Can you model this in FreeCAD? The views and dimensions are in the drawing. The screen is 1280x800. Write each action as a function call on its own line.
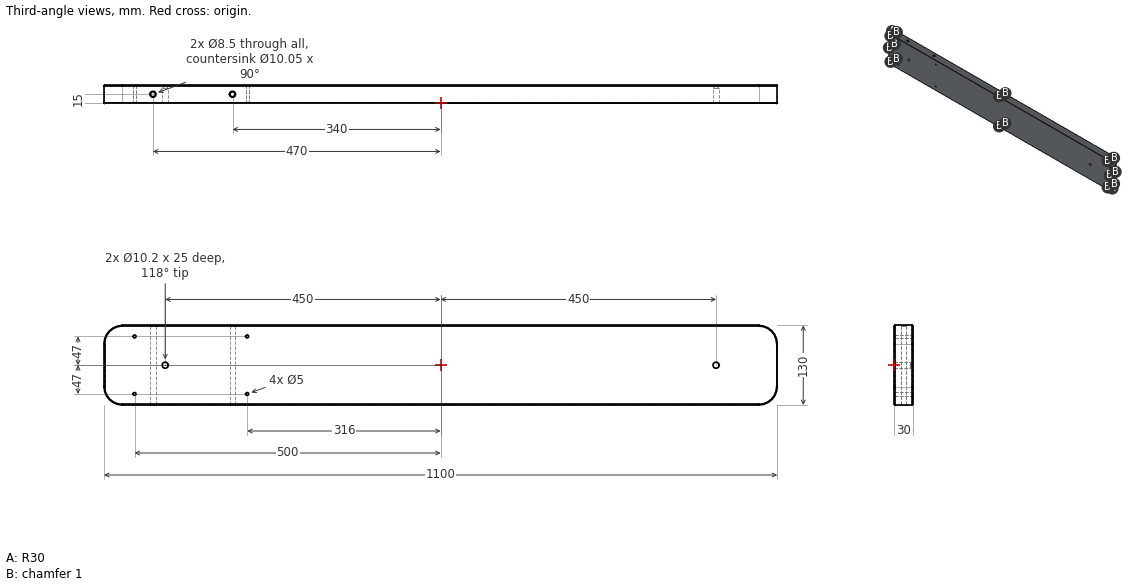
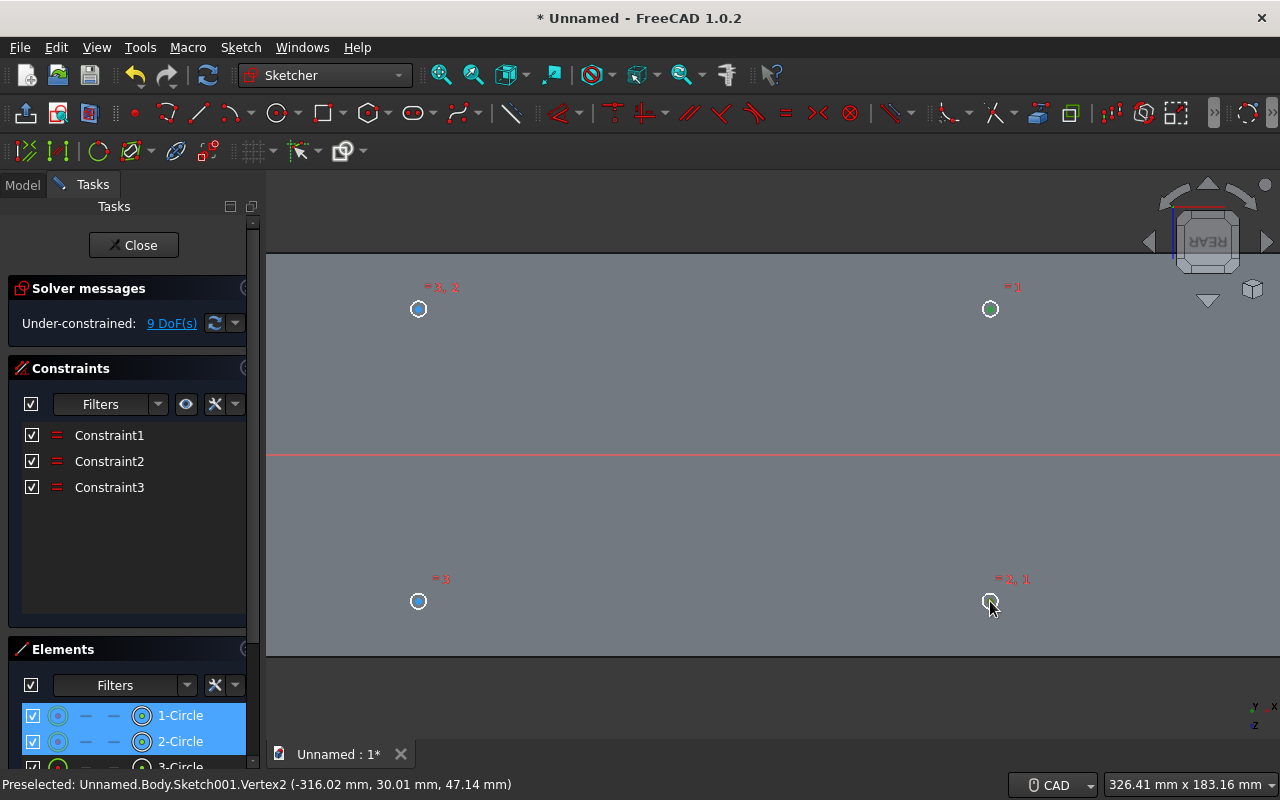
click(668, 114)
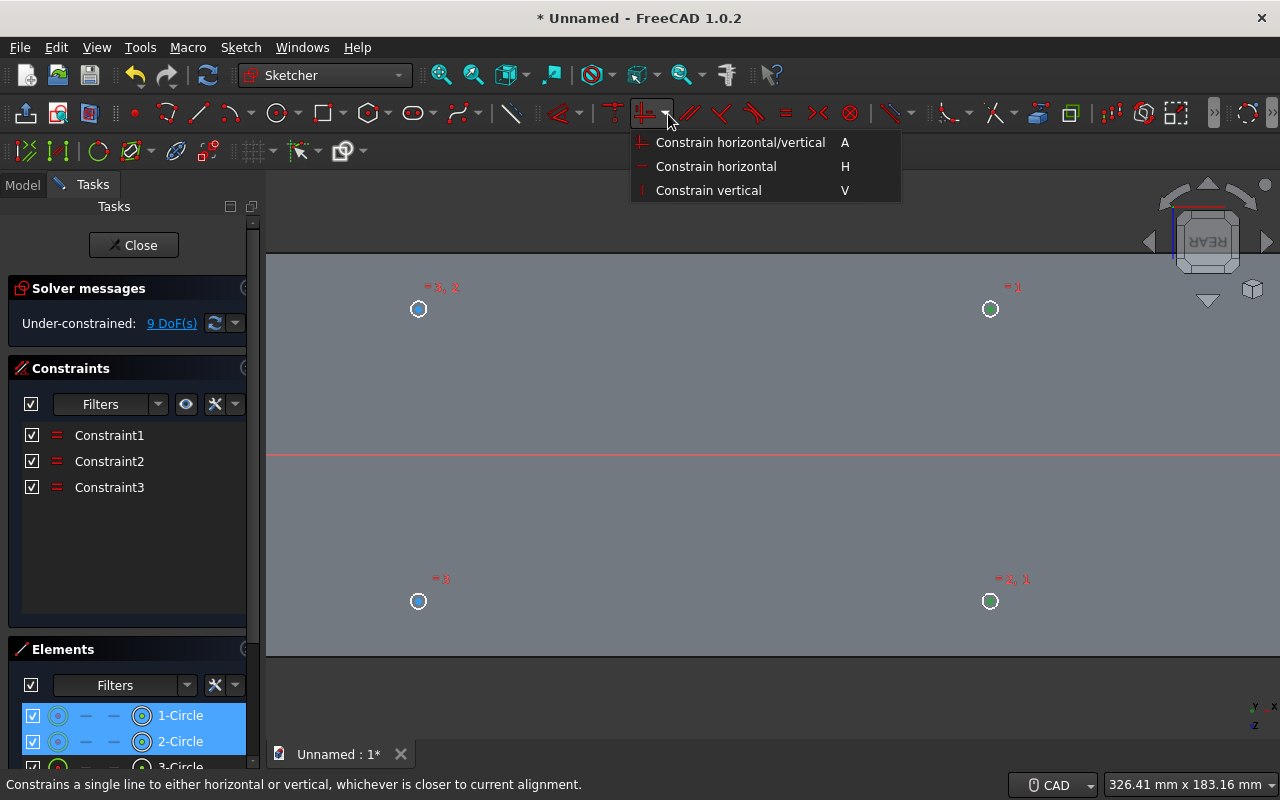
click(766, 190)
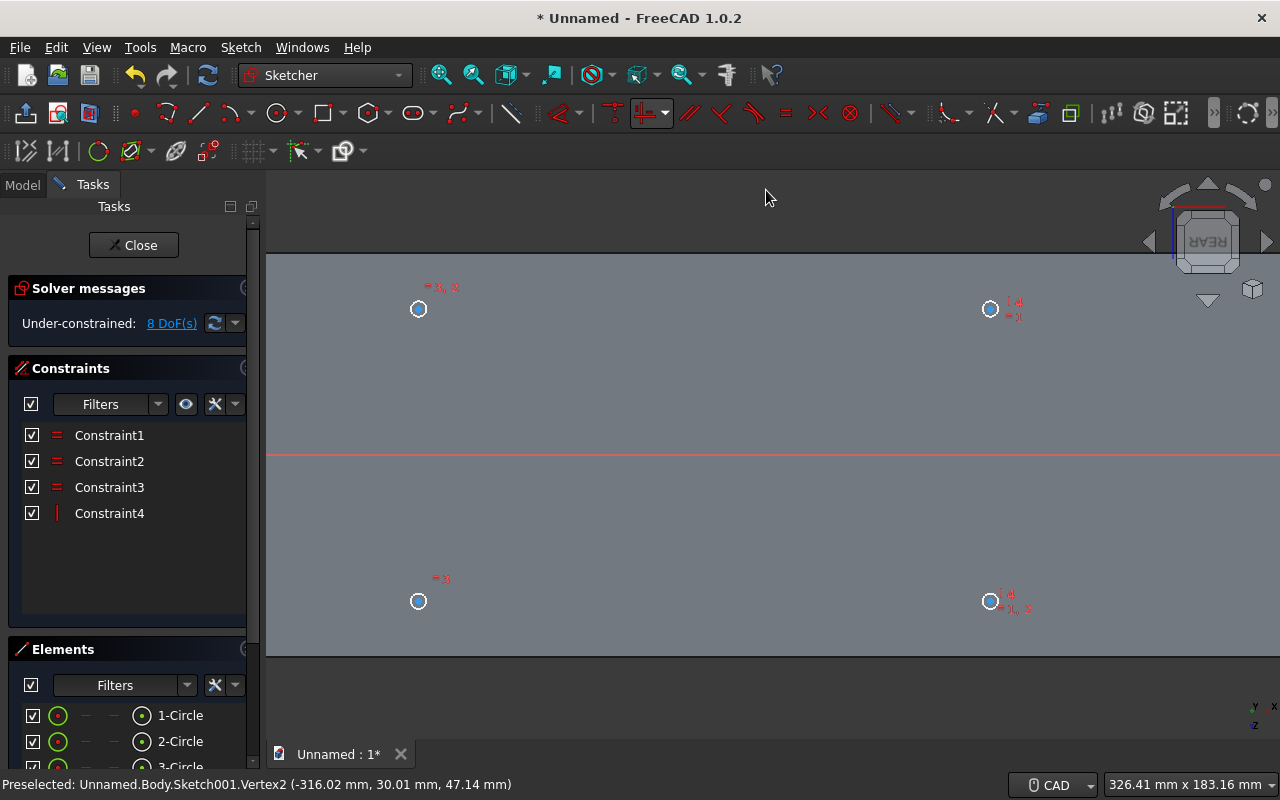
click(990, 309)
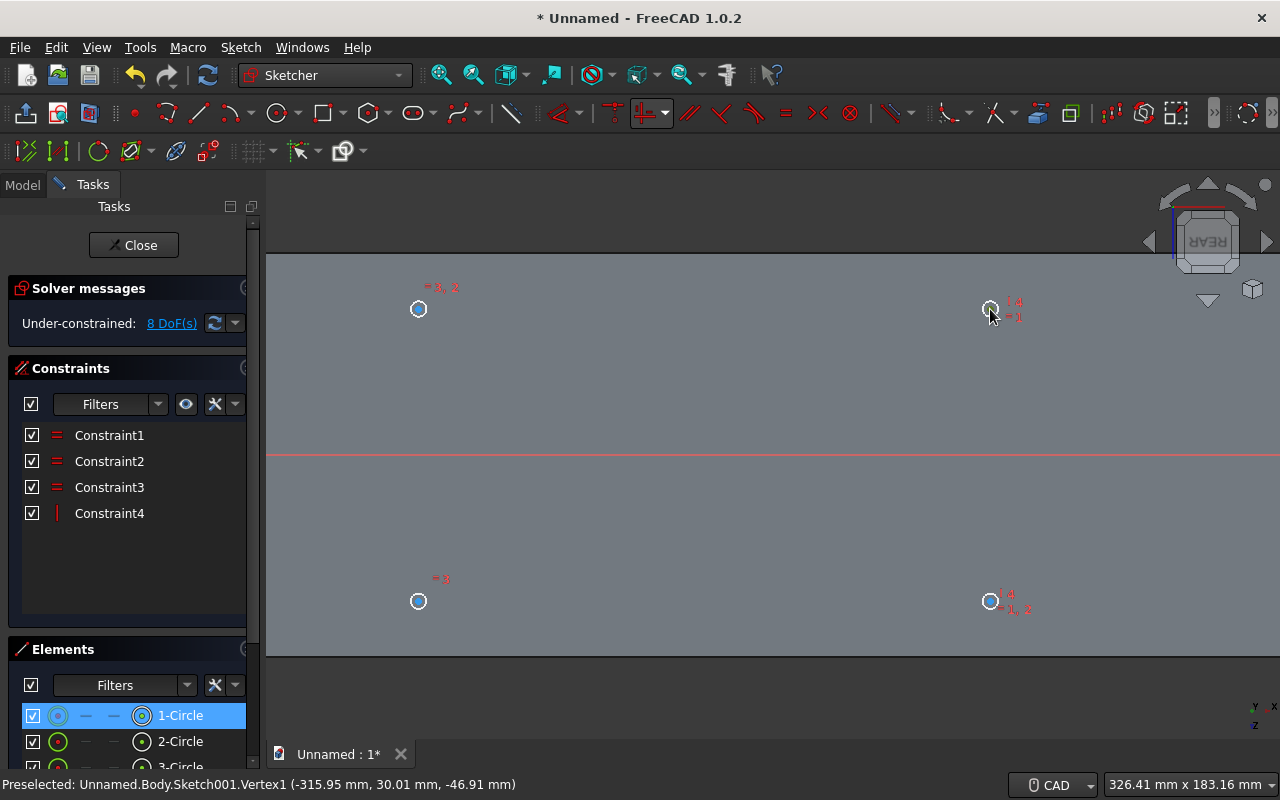
click(419, 309)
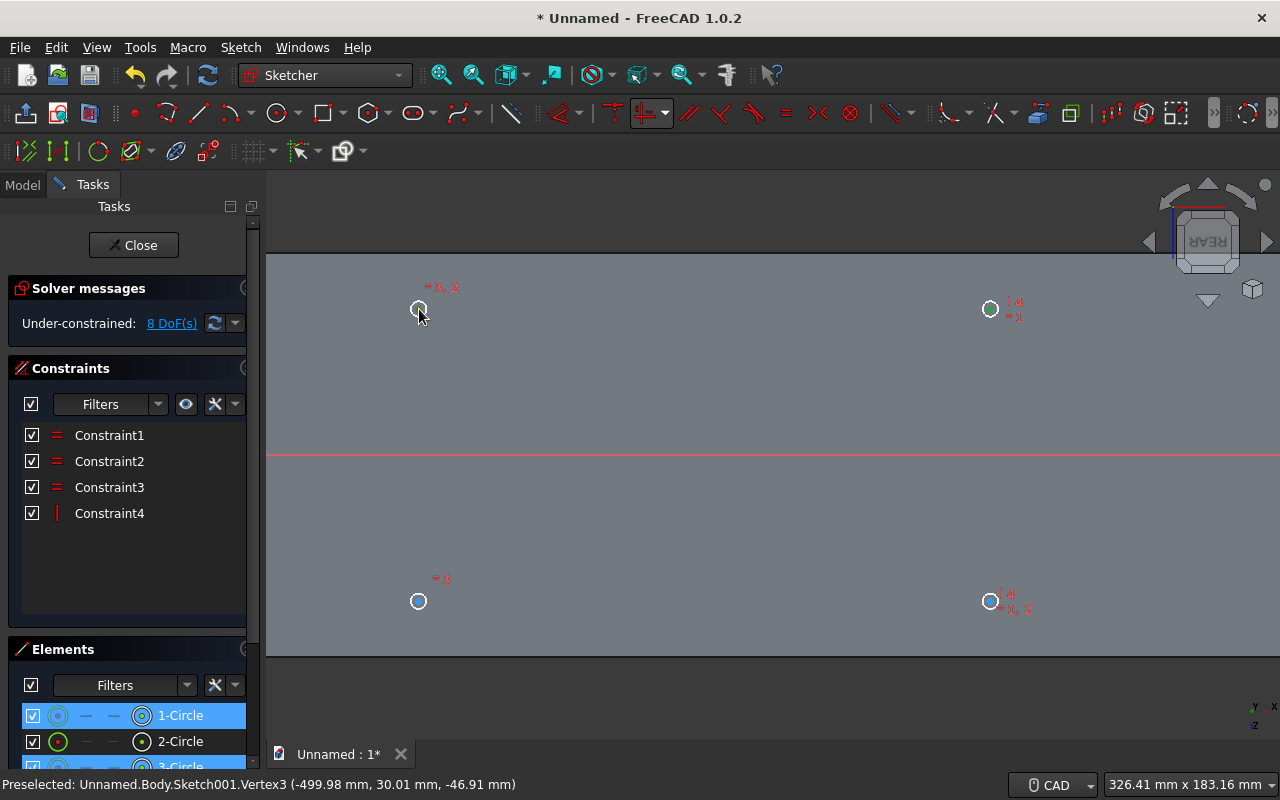
click(668, 114)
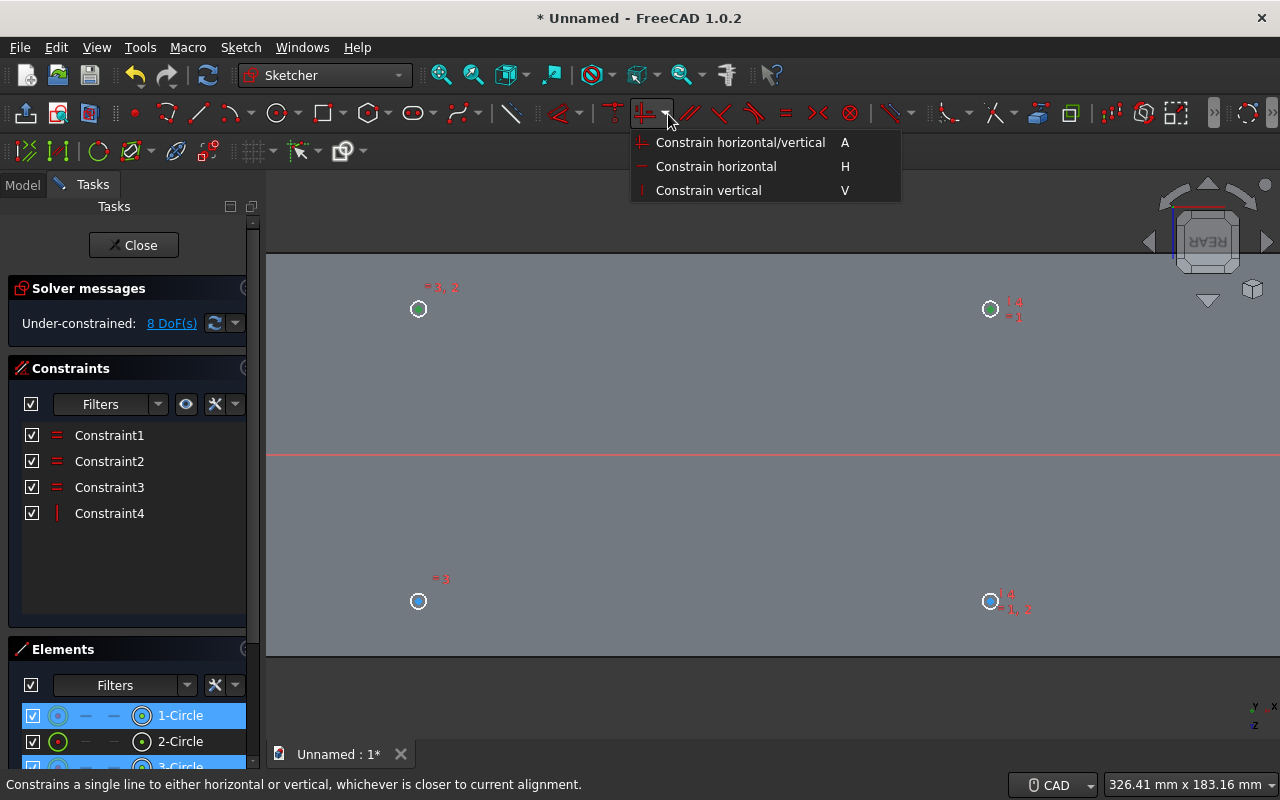
click(766, 166)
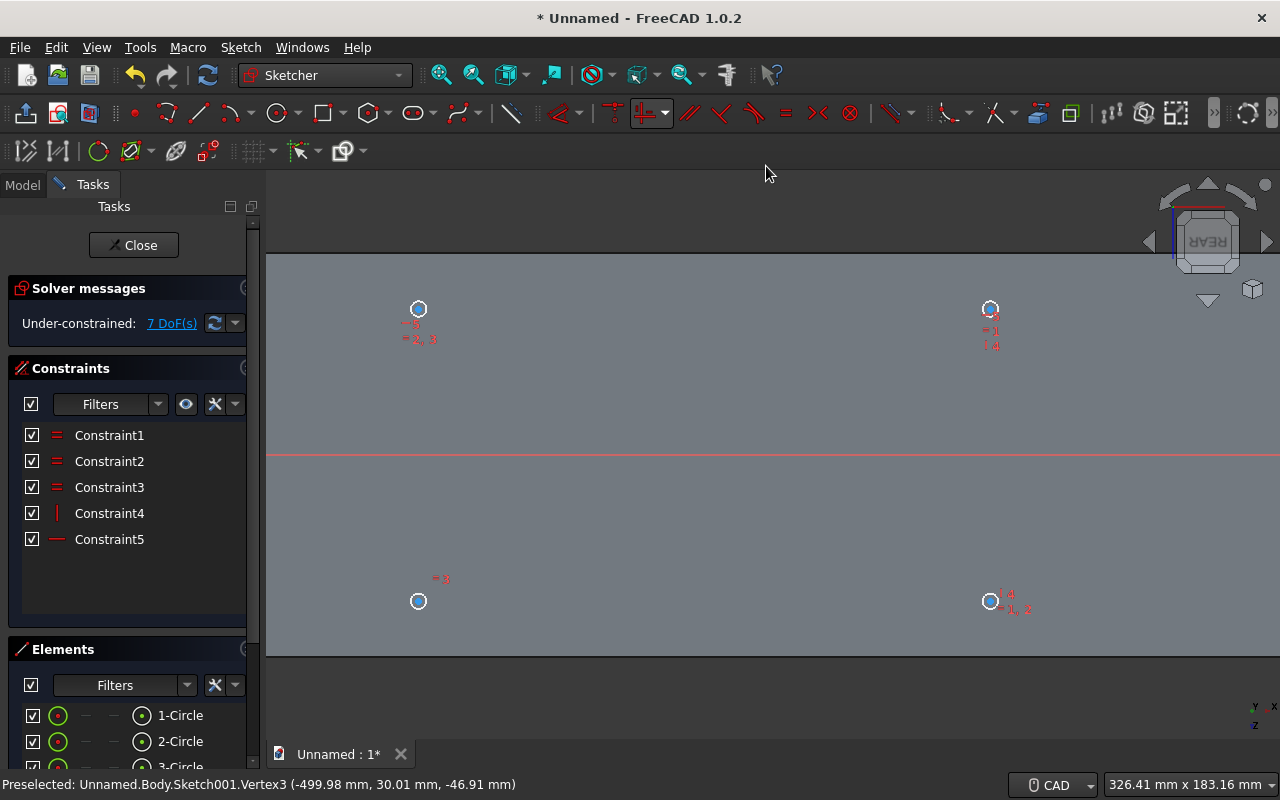
click(419, 309)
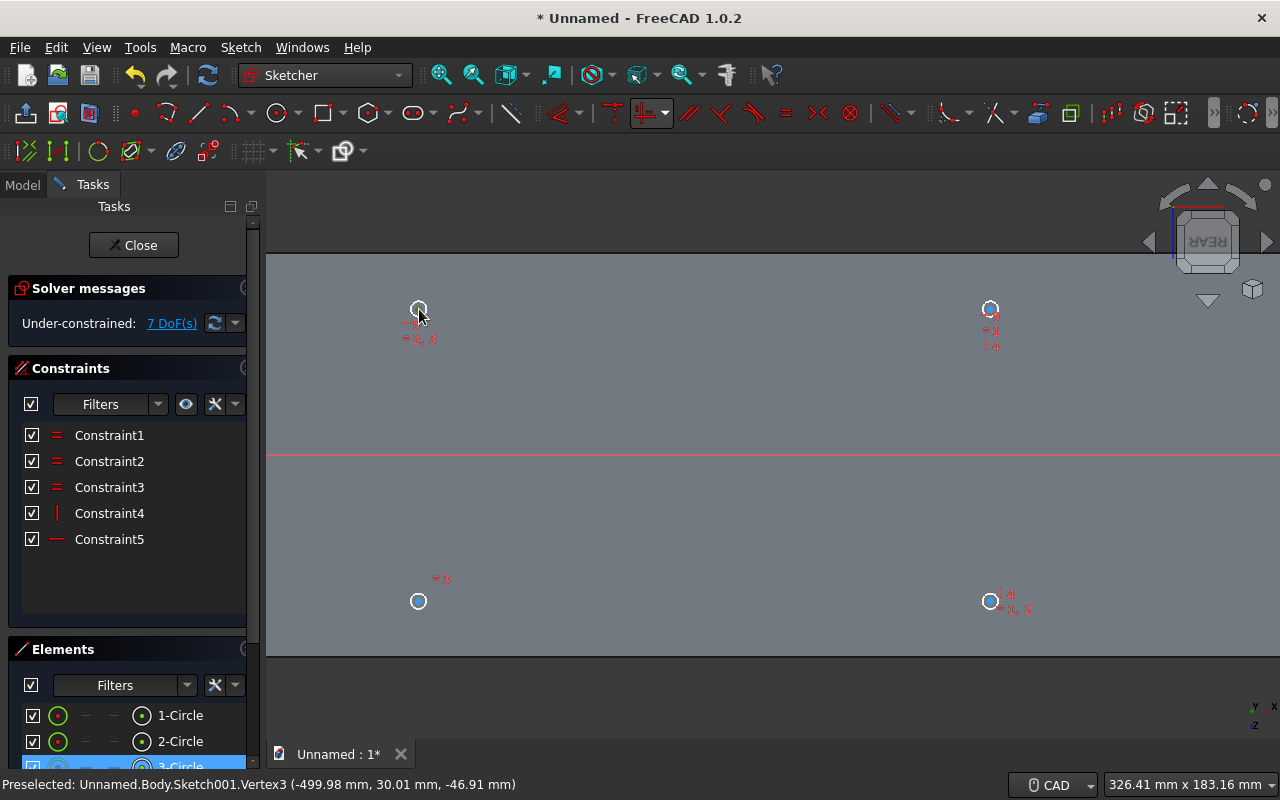
click(419, 601)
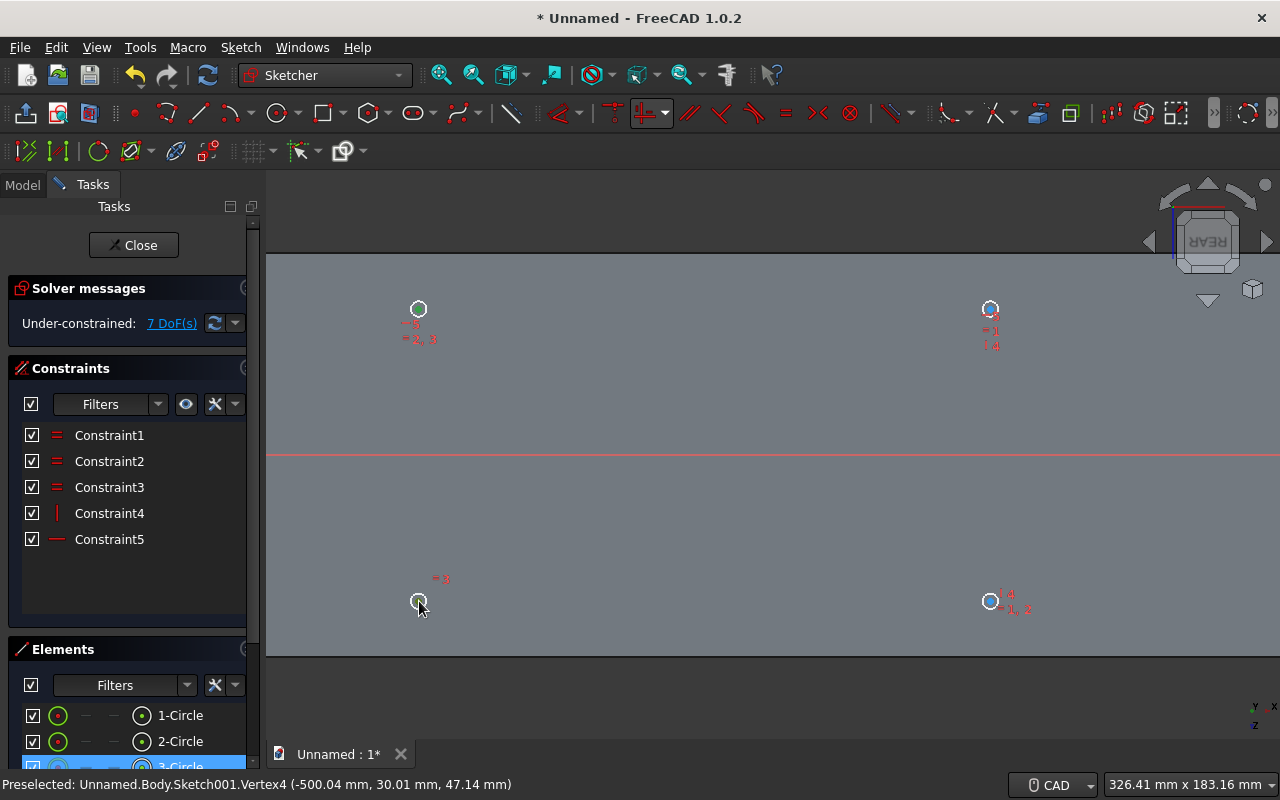
key(v)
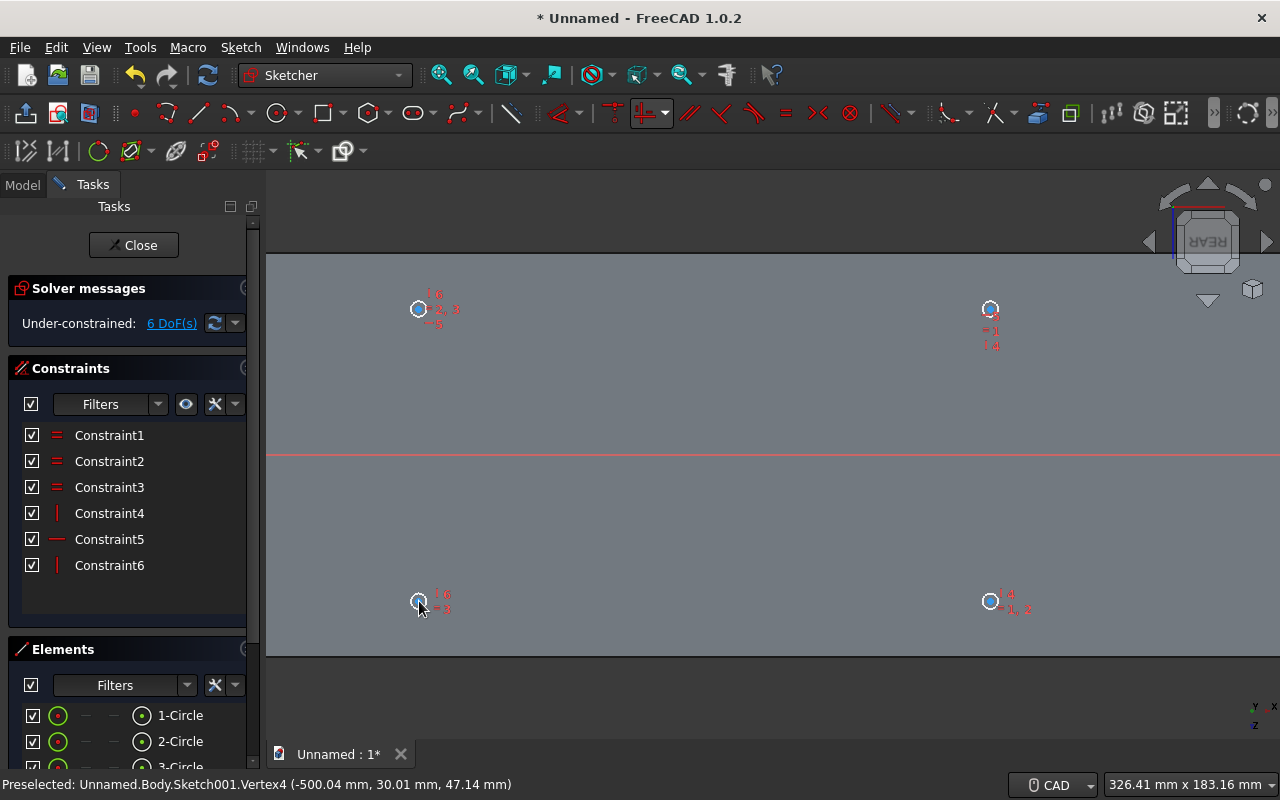
click(990, 601)